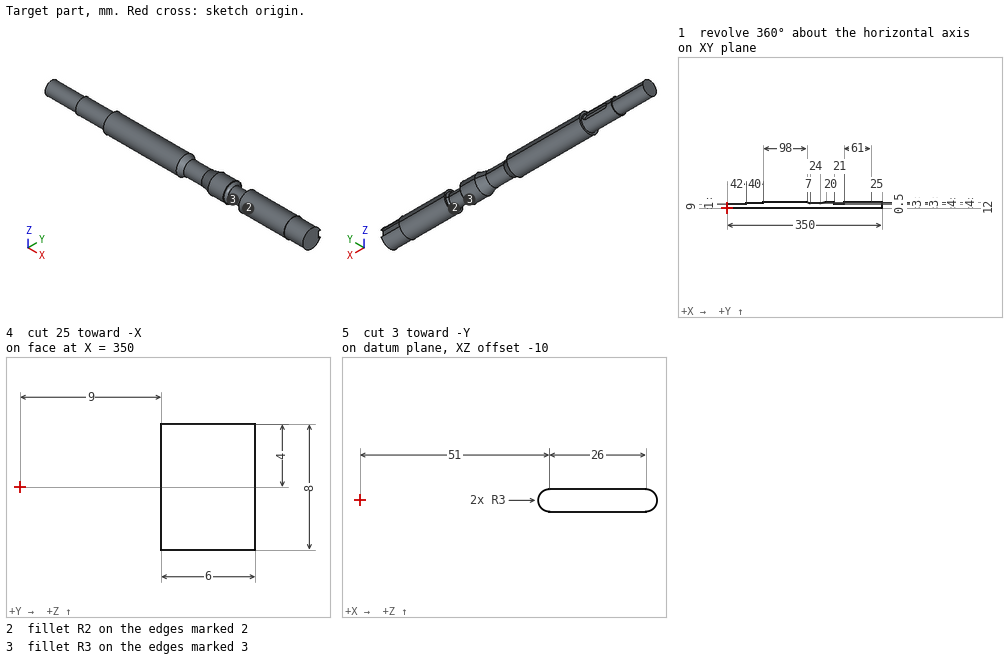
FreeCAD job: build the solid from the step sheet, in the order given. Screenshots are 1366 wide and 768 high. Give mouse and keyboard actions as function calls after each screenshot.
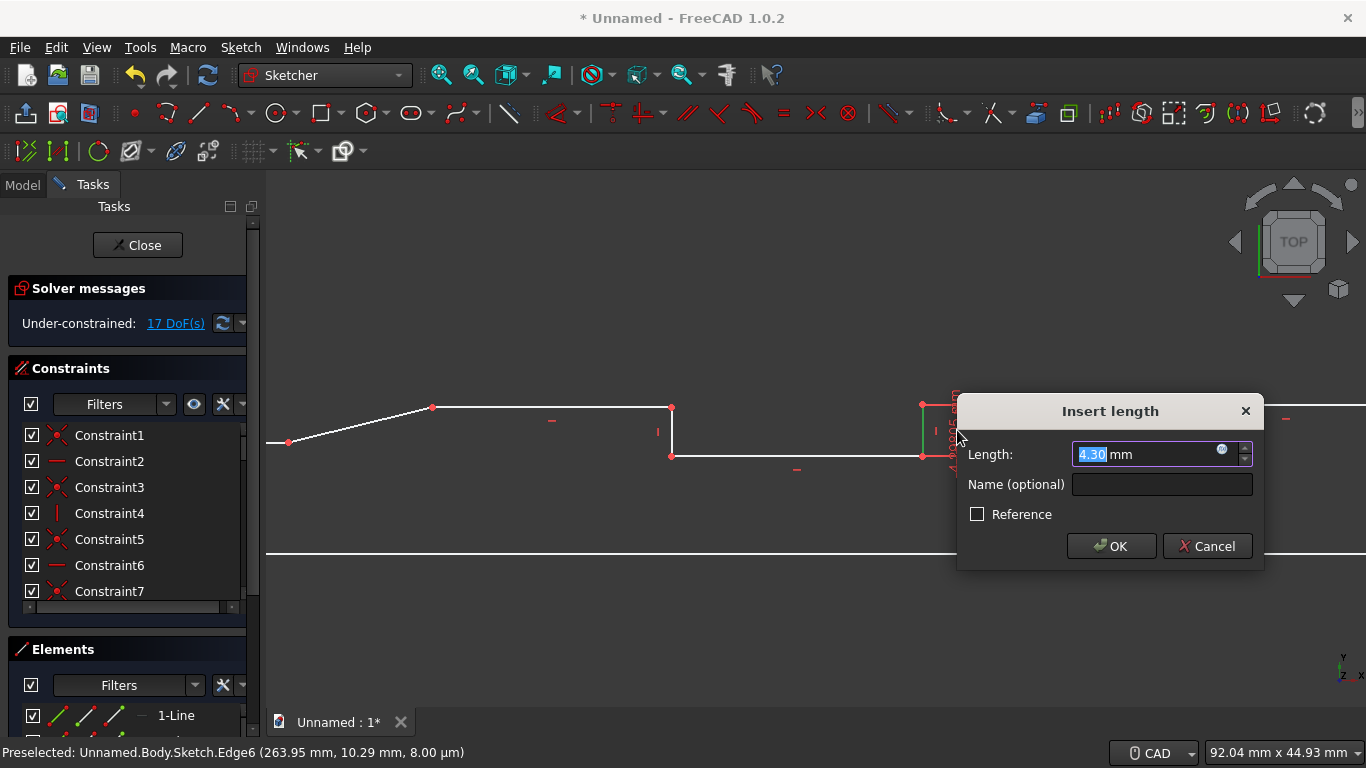
text(4)
key(Return)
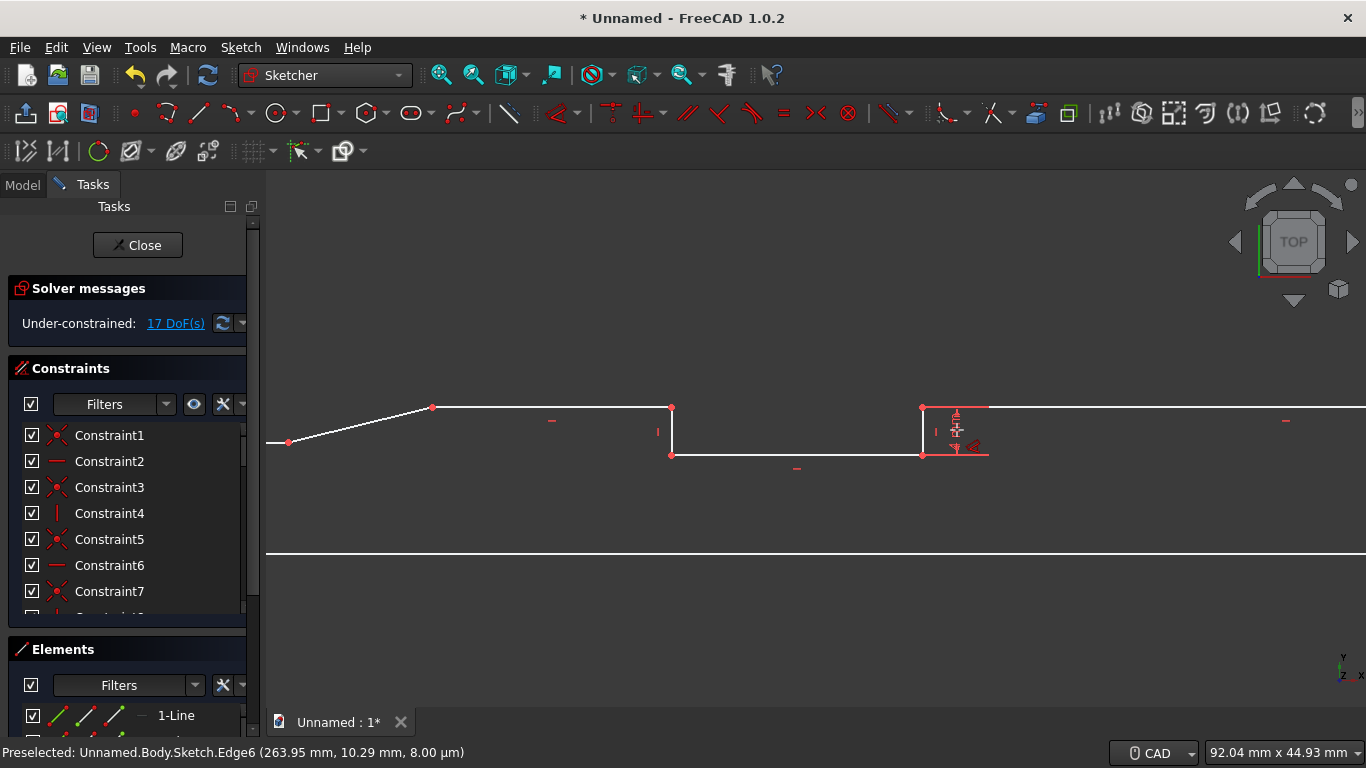
click(672, 441)
click(706, 431)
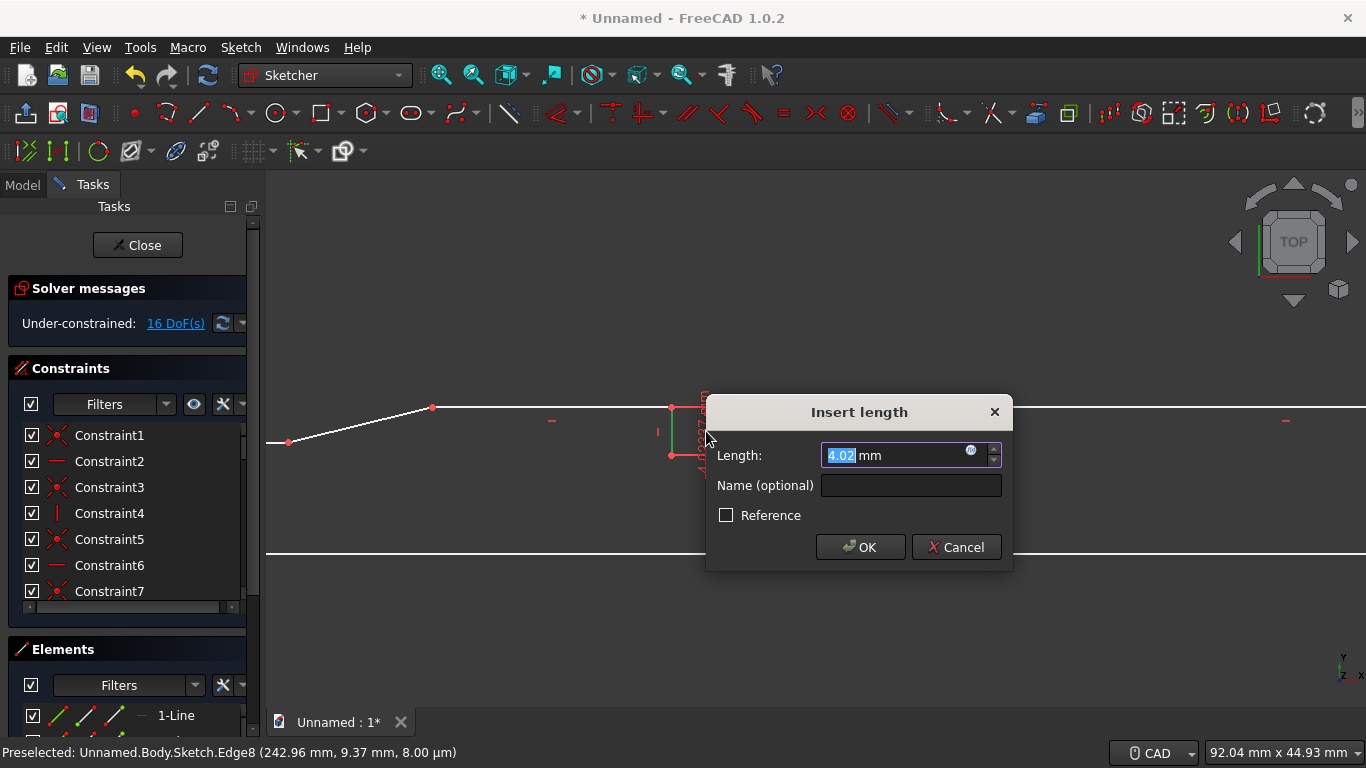
text(4)
key(Return)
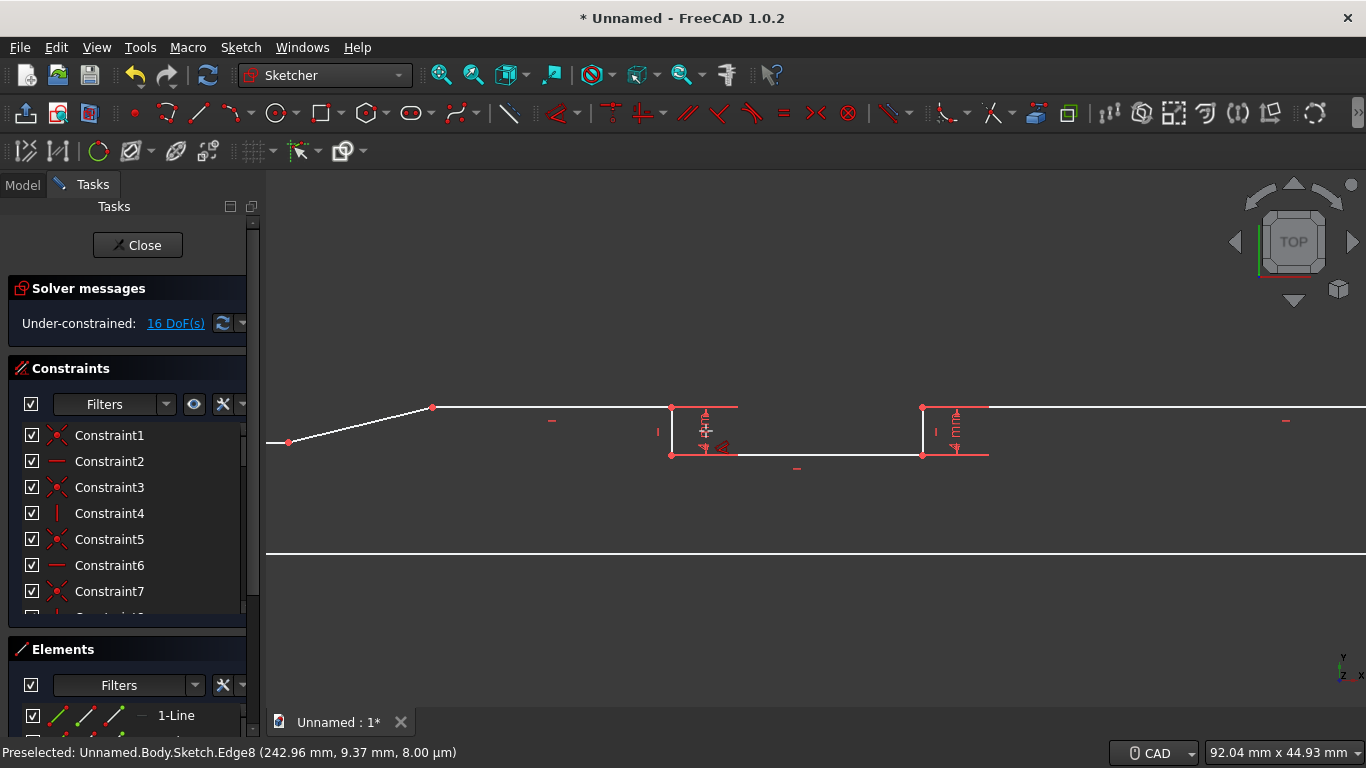
scroll(923, 430, down, 9)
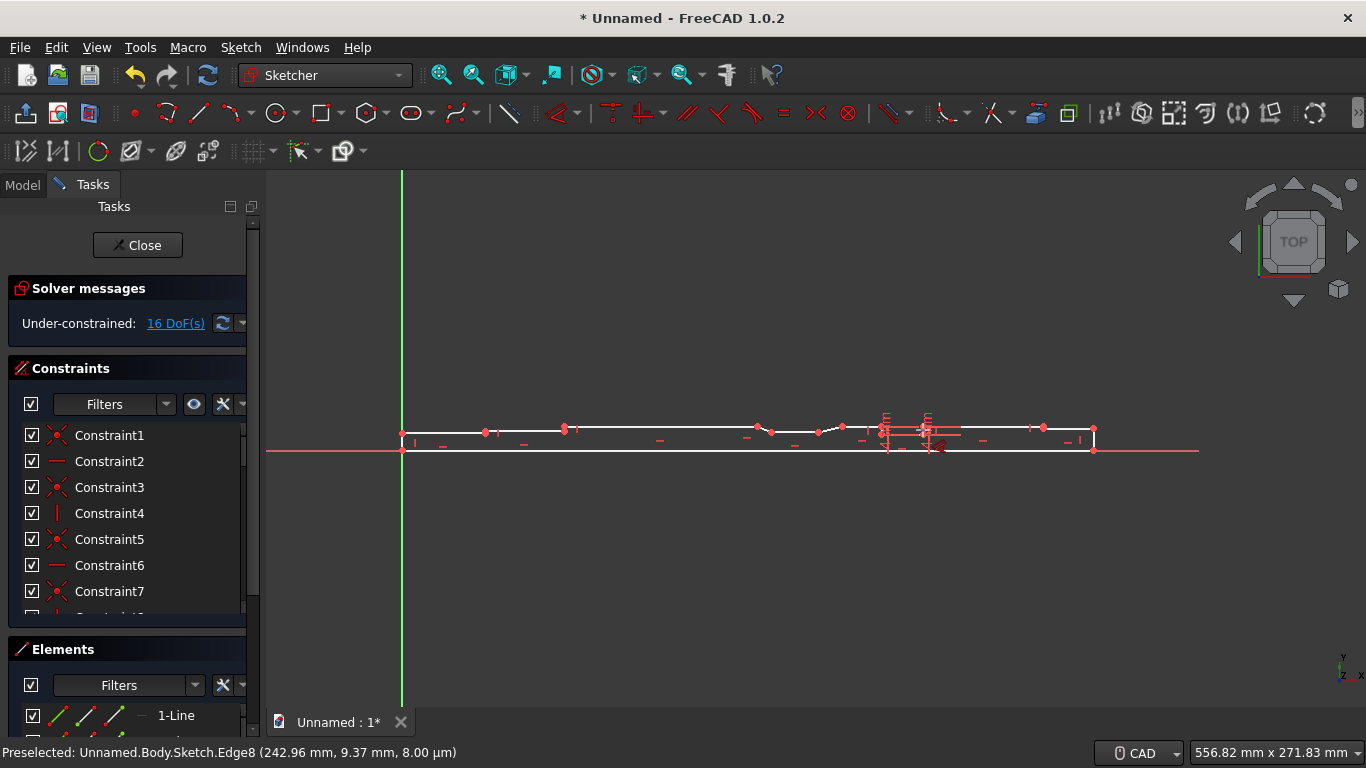
scroll(485, 432, up, 16)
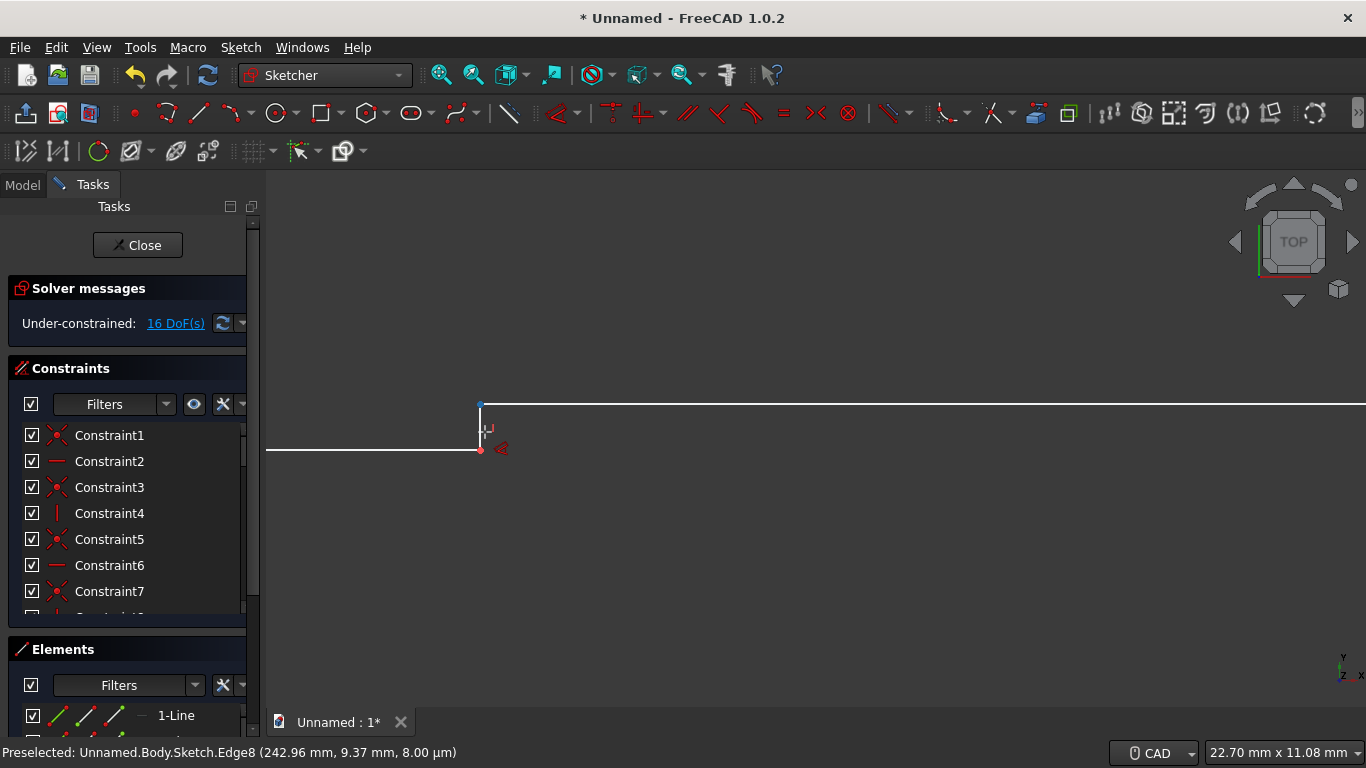
click(480, 427)
click(446, 427)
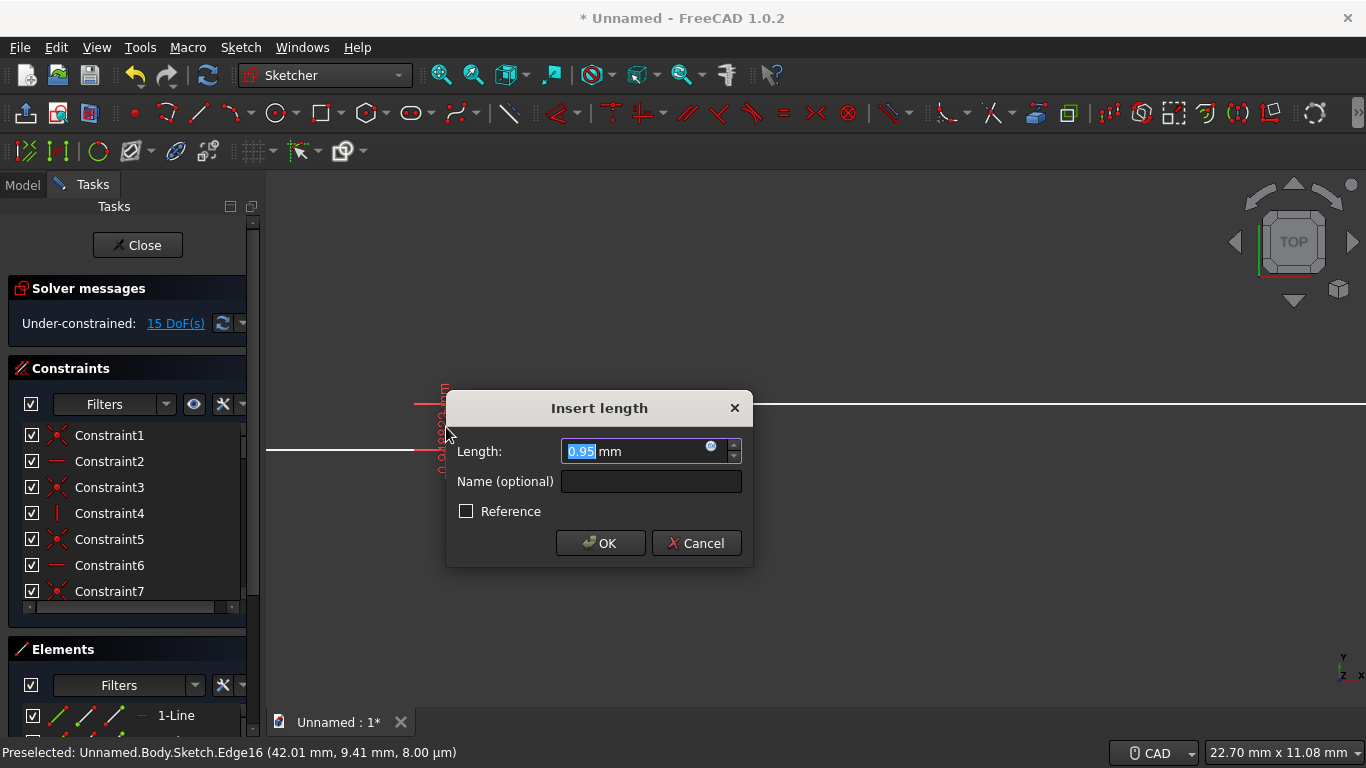
text(1)
key(Return)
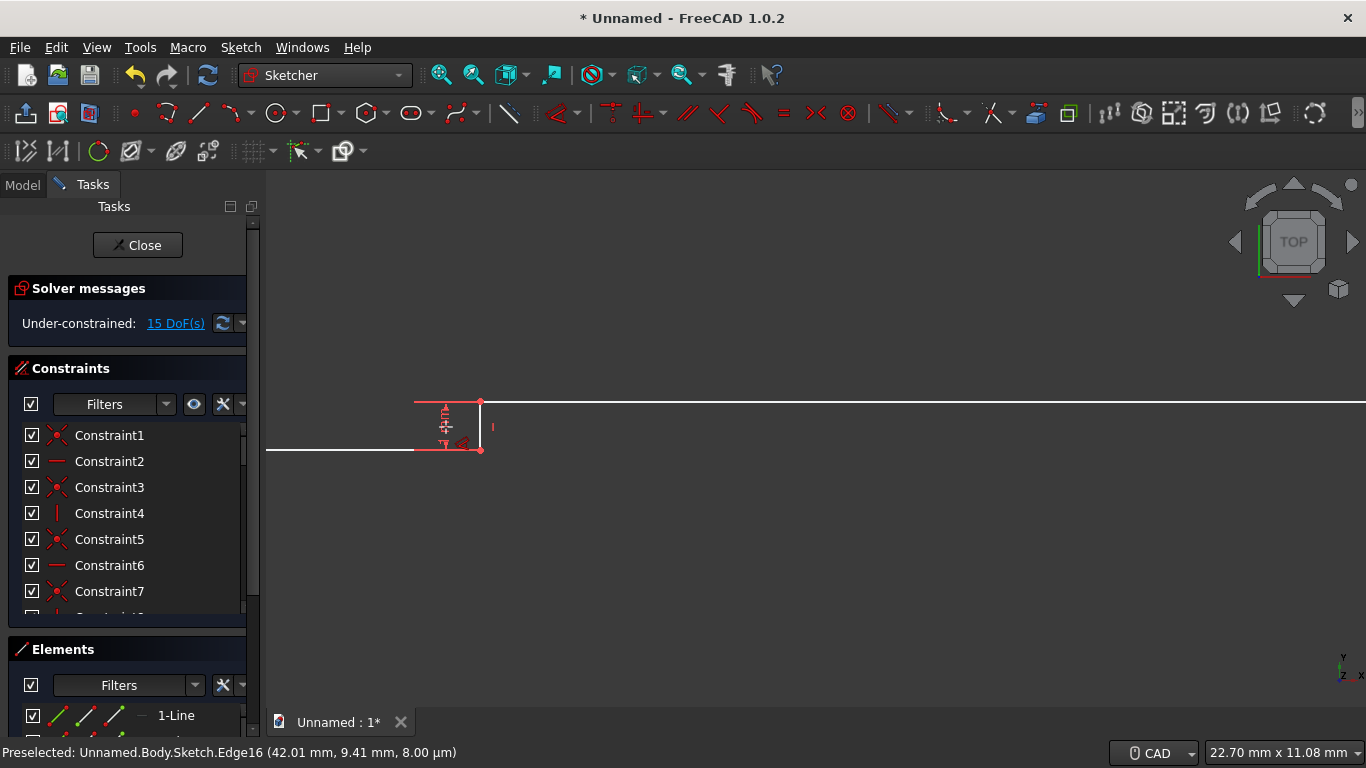
scroll(424, 431, down, 15)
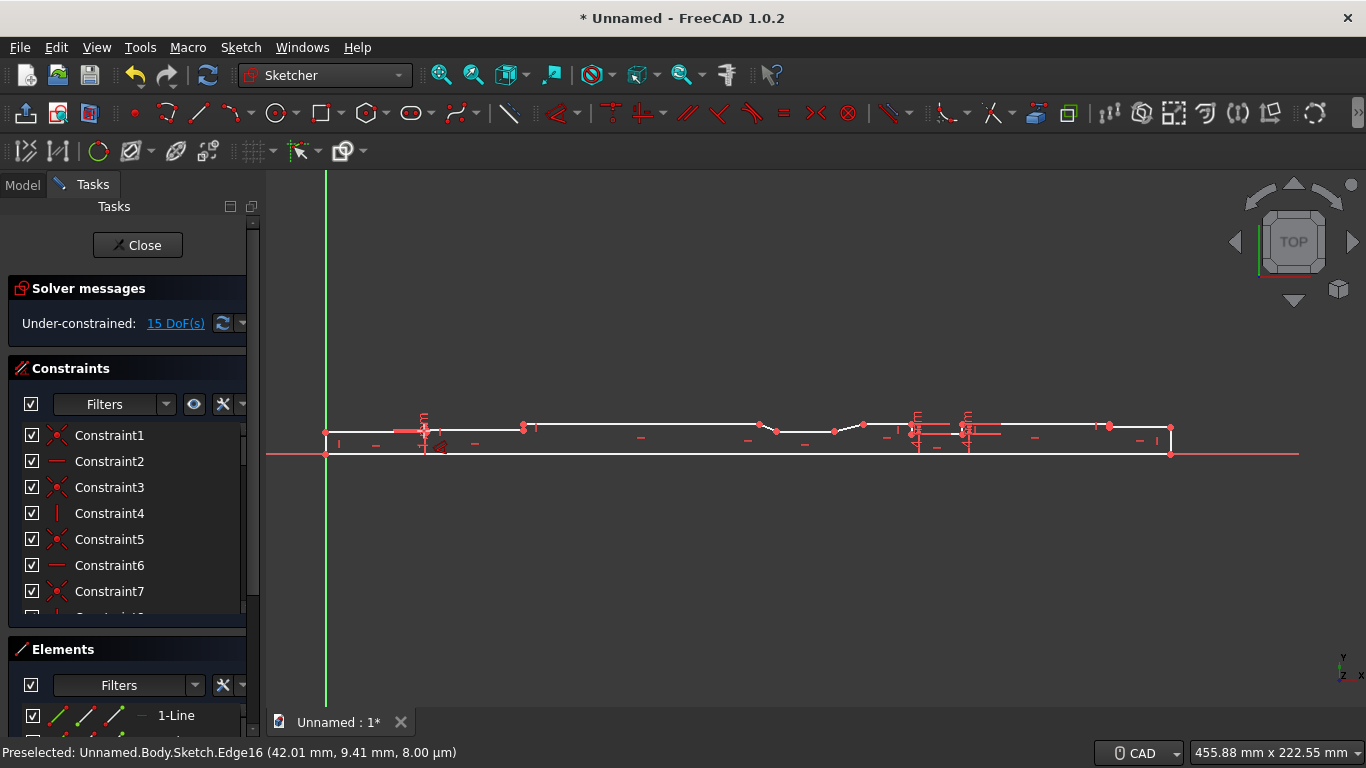
scroll(326, 439, up, 4)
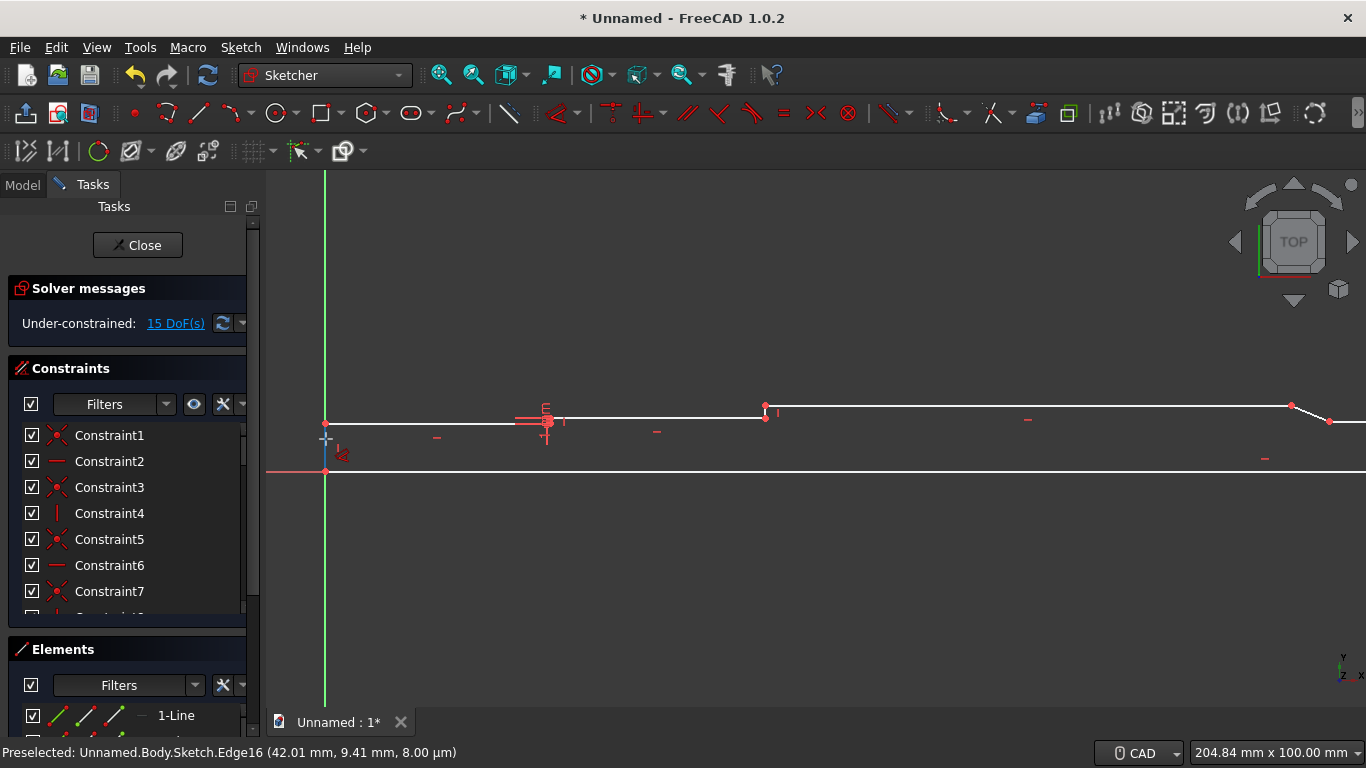
click(325, 438)
click(359, 448)